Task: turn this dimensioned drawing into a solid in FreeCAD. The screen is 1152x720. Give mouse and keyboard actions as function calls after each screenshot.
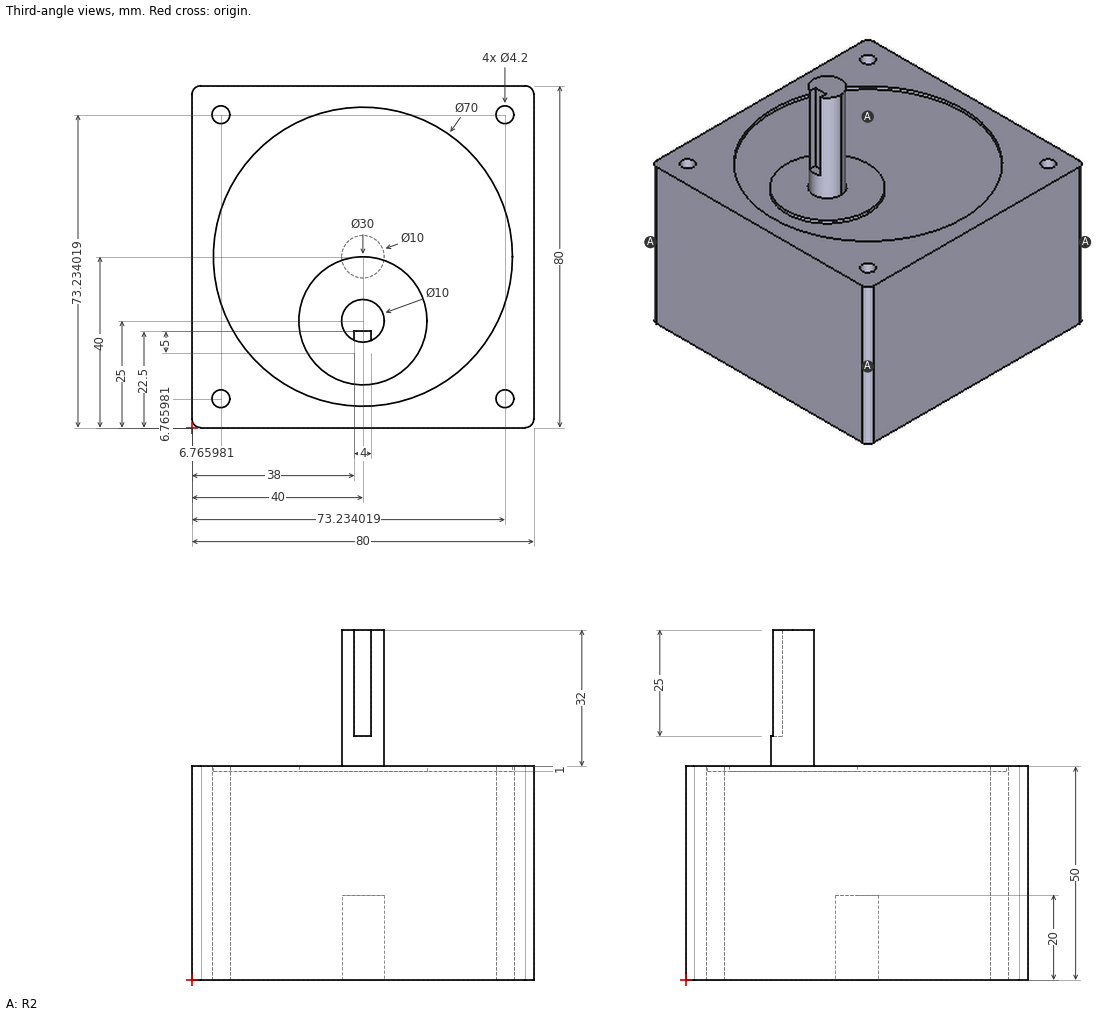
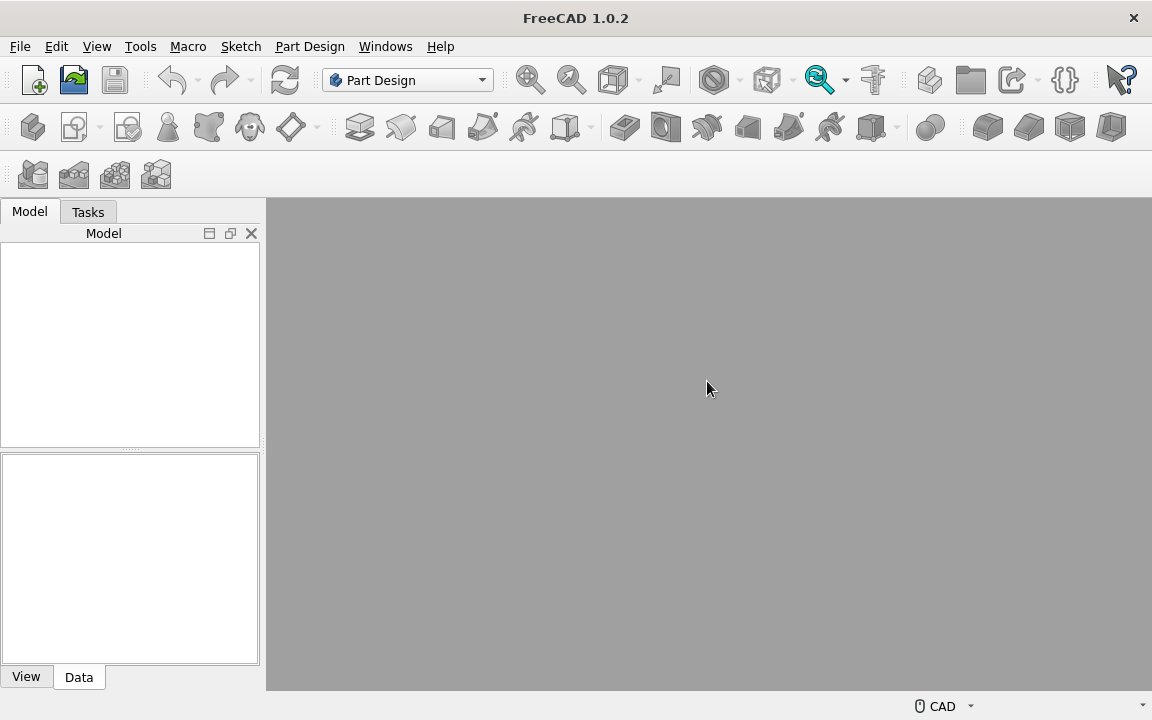
key(ctrl+n)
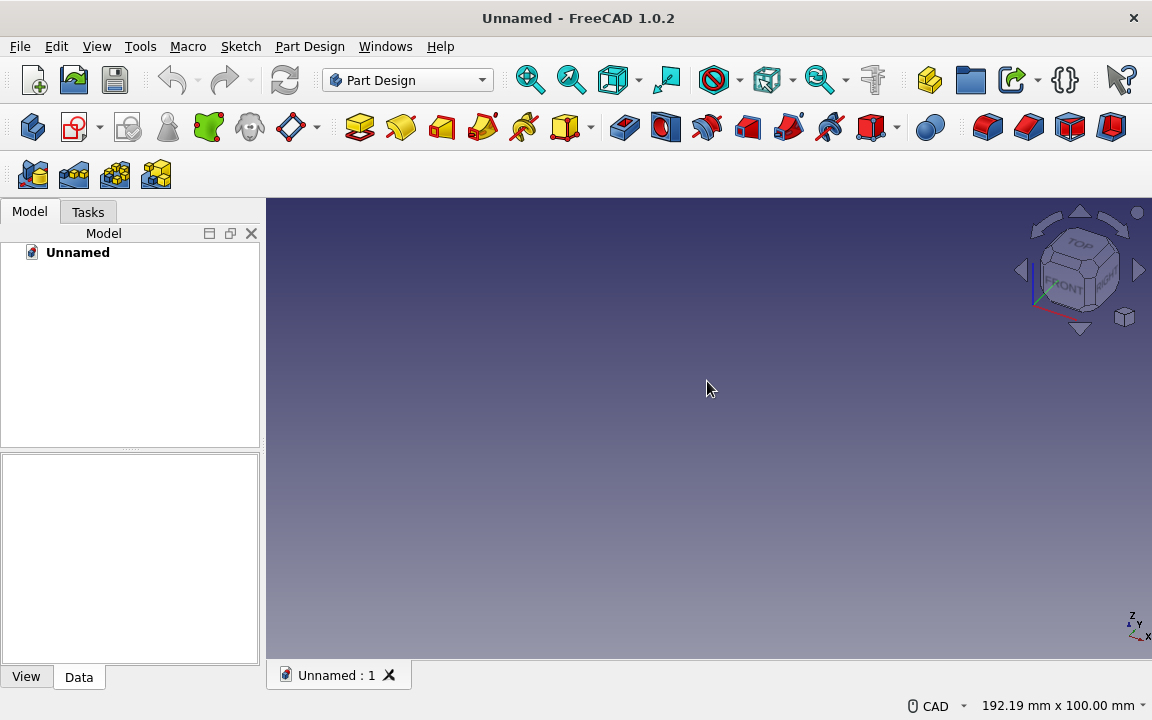
click(74, 128)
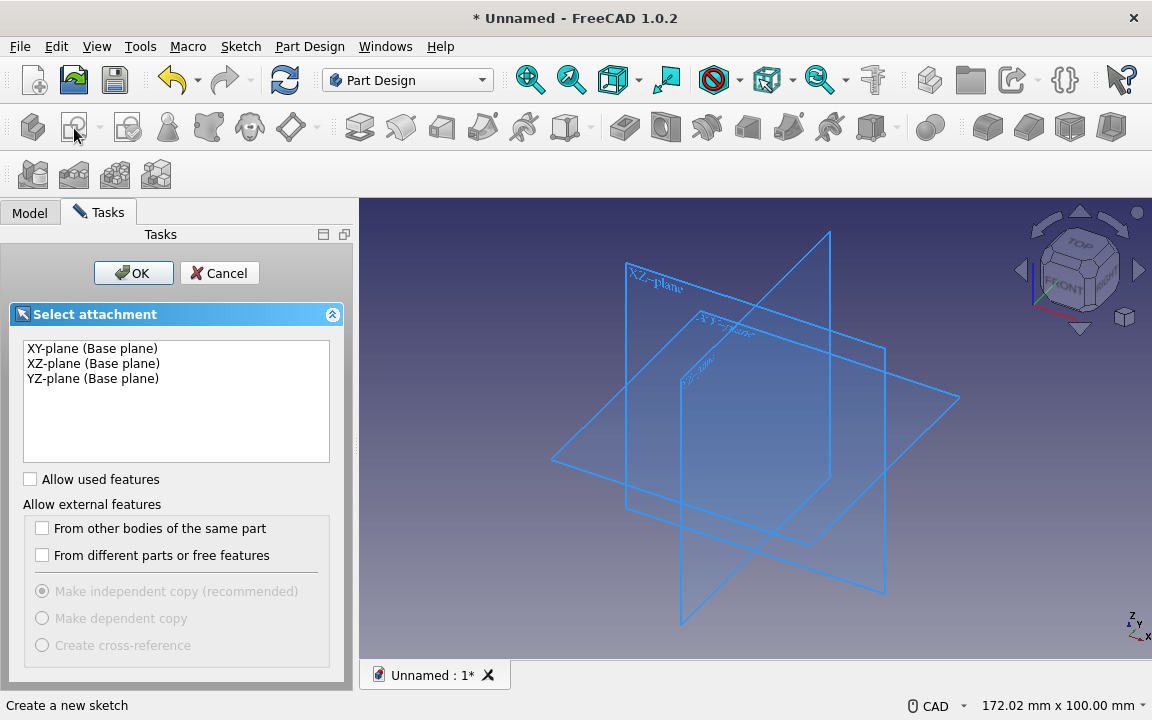
click(84, 348)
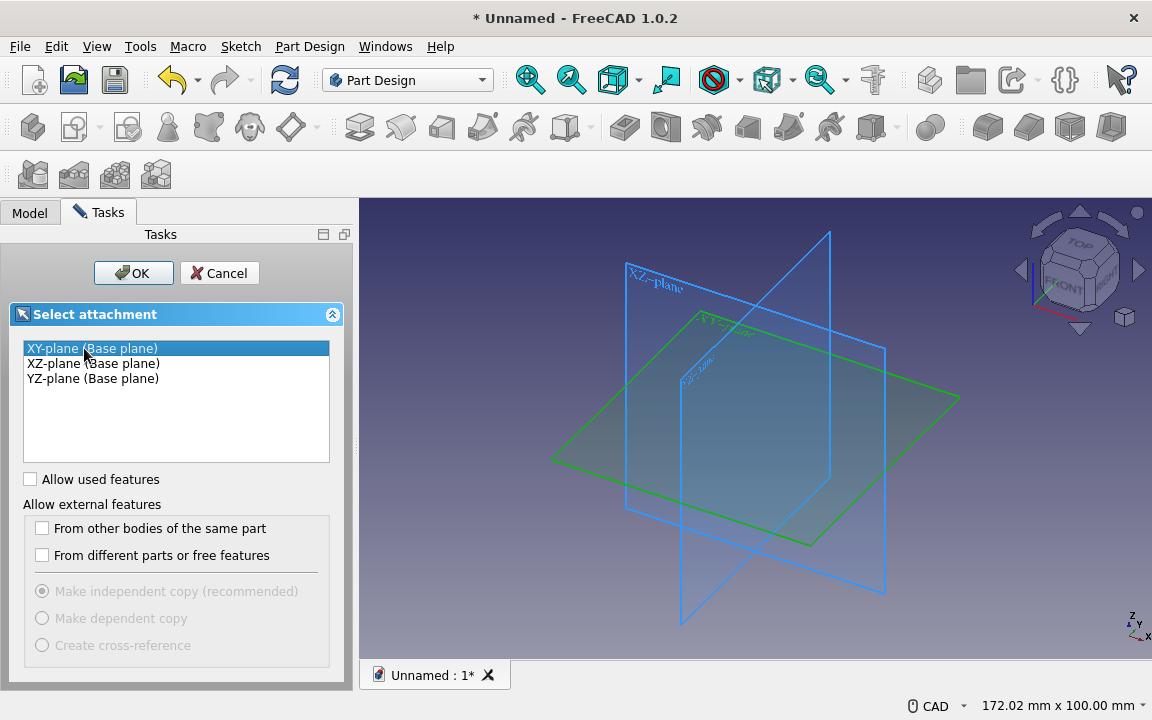
click(134, 273)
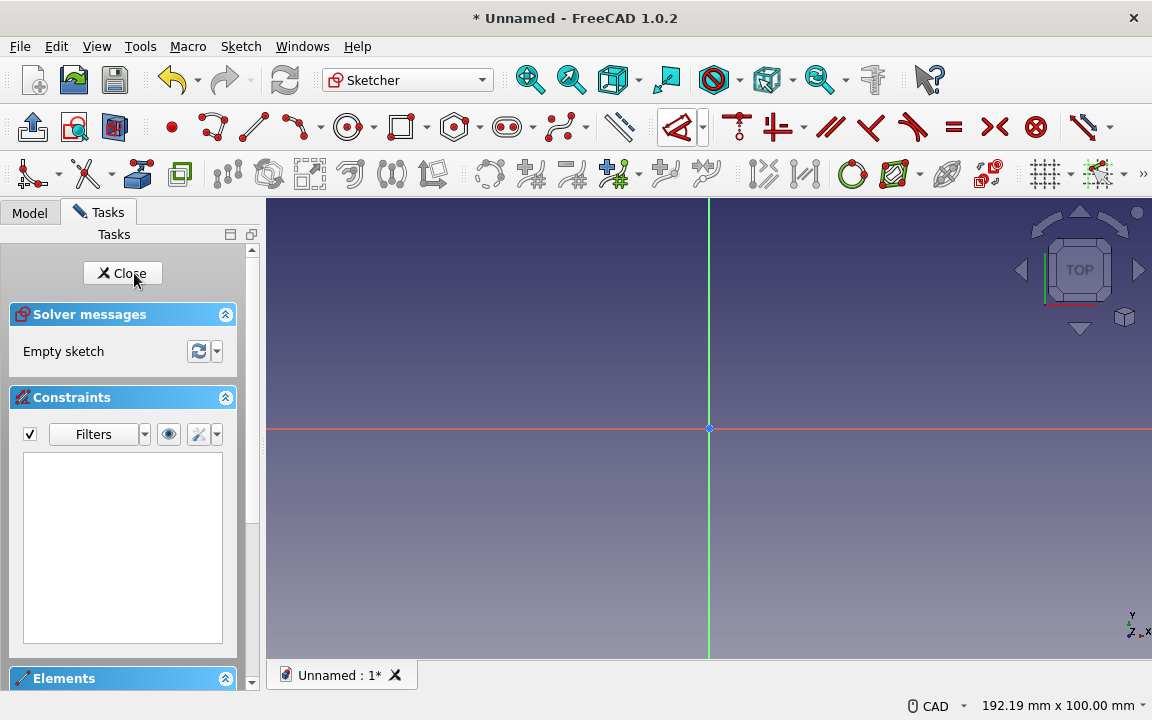
scroll(333, 631, down, 3)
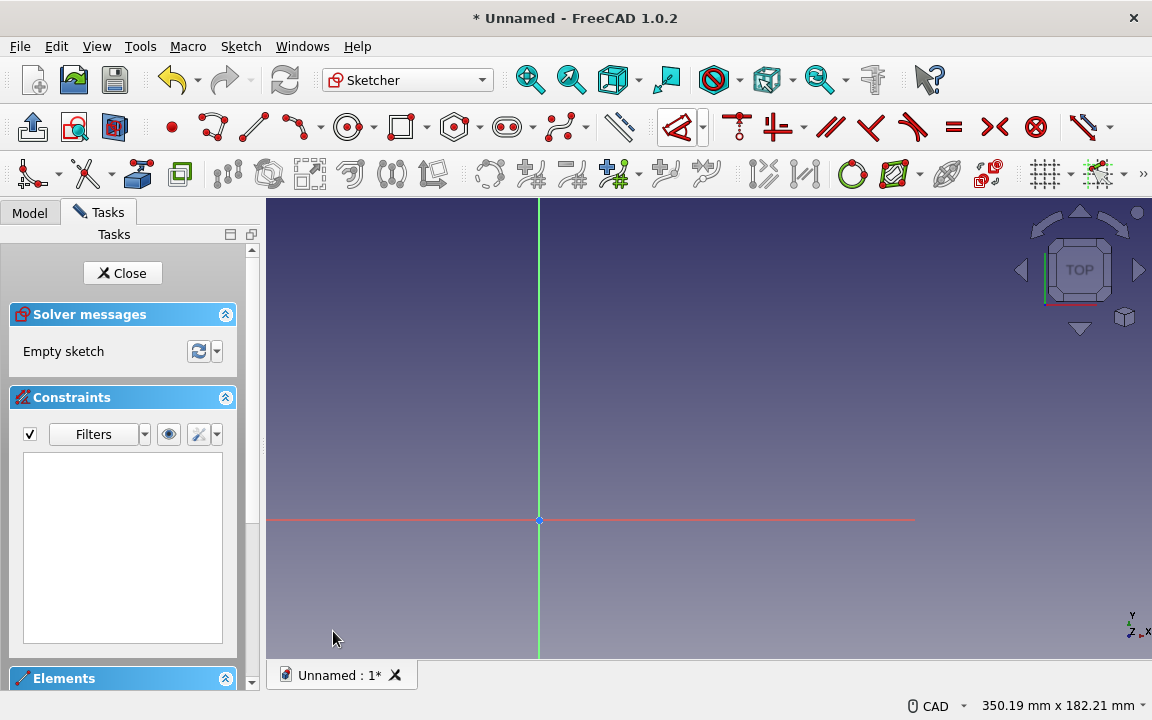
scroll(641, 400, up, 2)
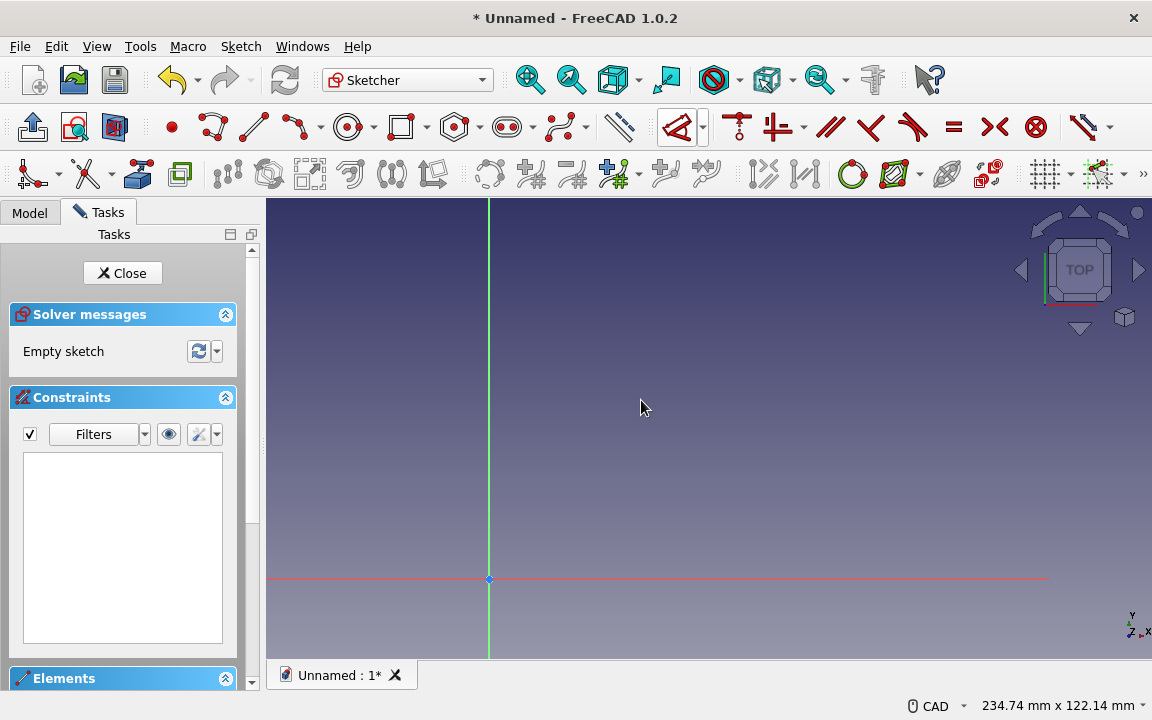
click(400, 128)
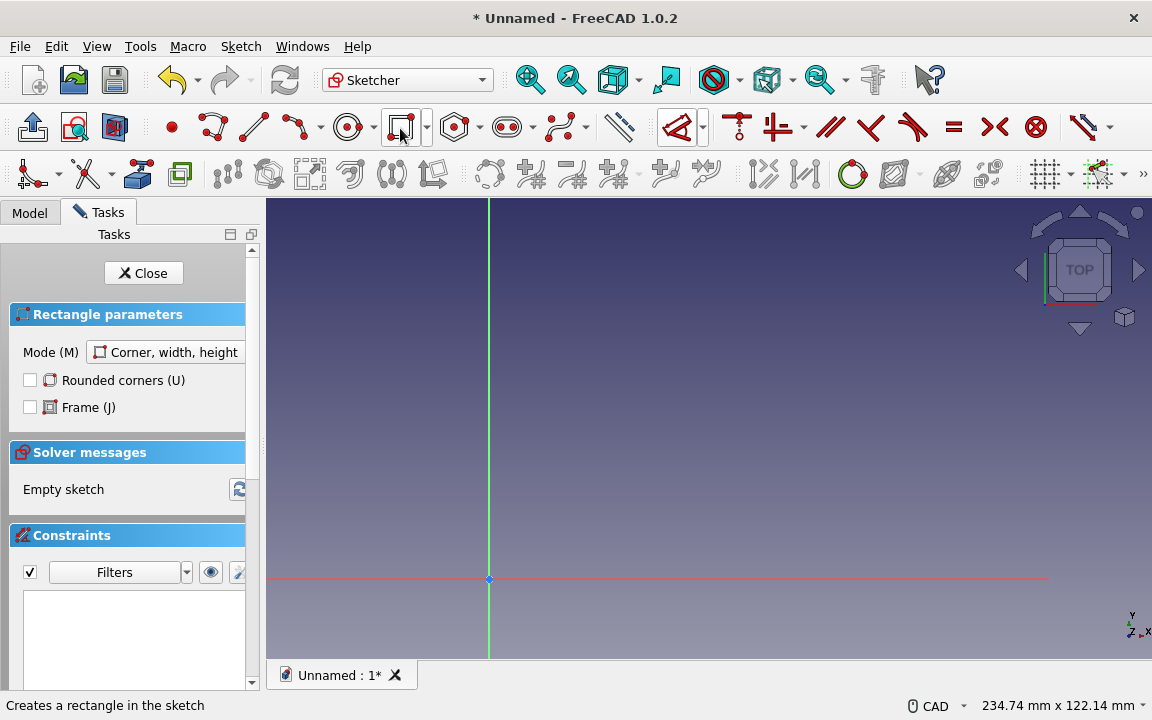
click(489, 579)
click(791, 277)
key(Escape)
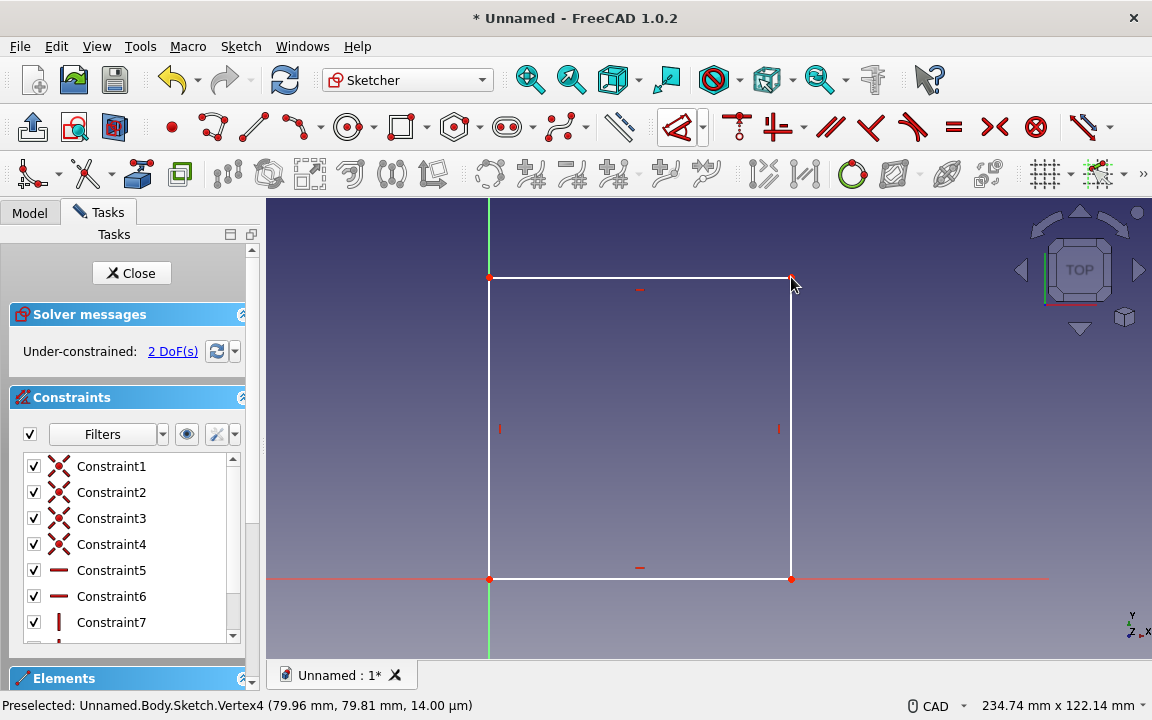
click(580, 579)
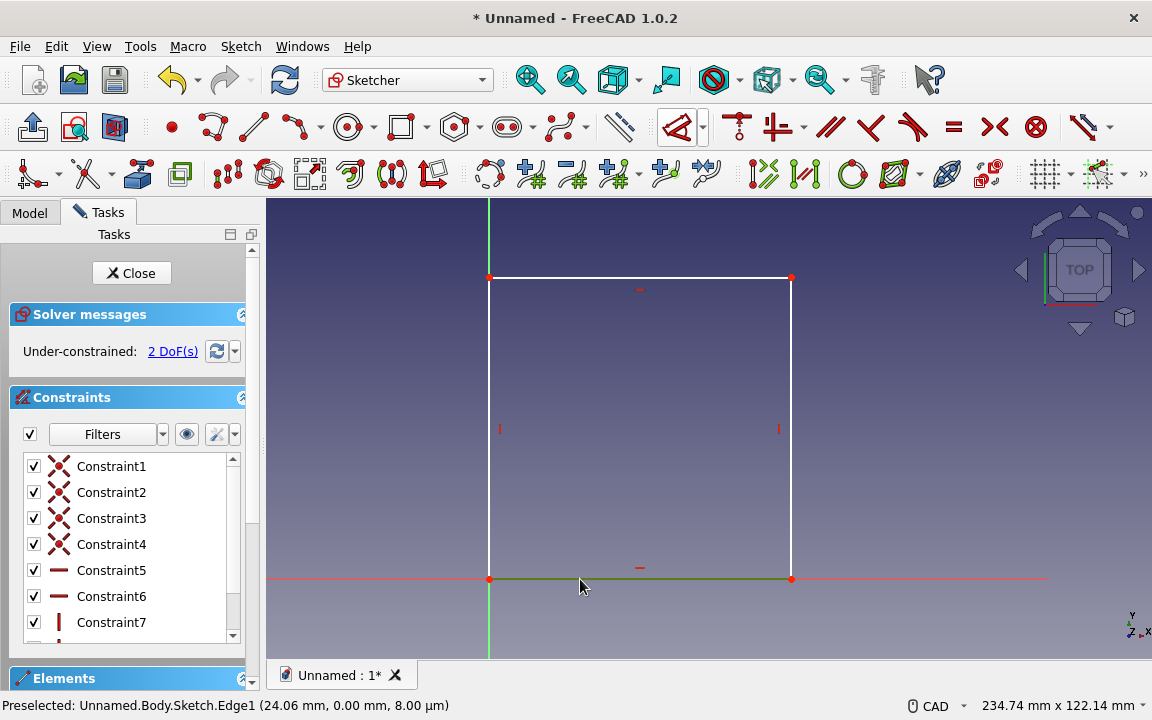
key(l)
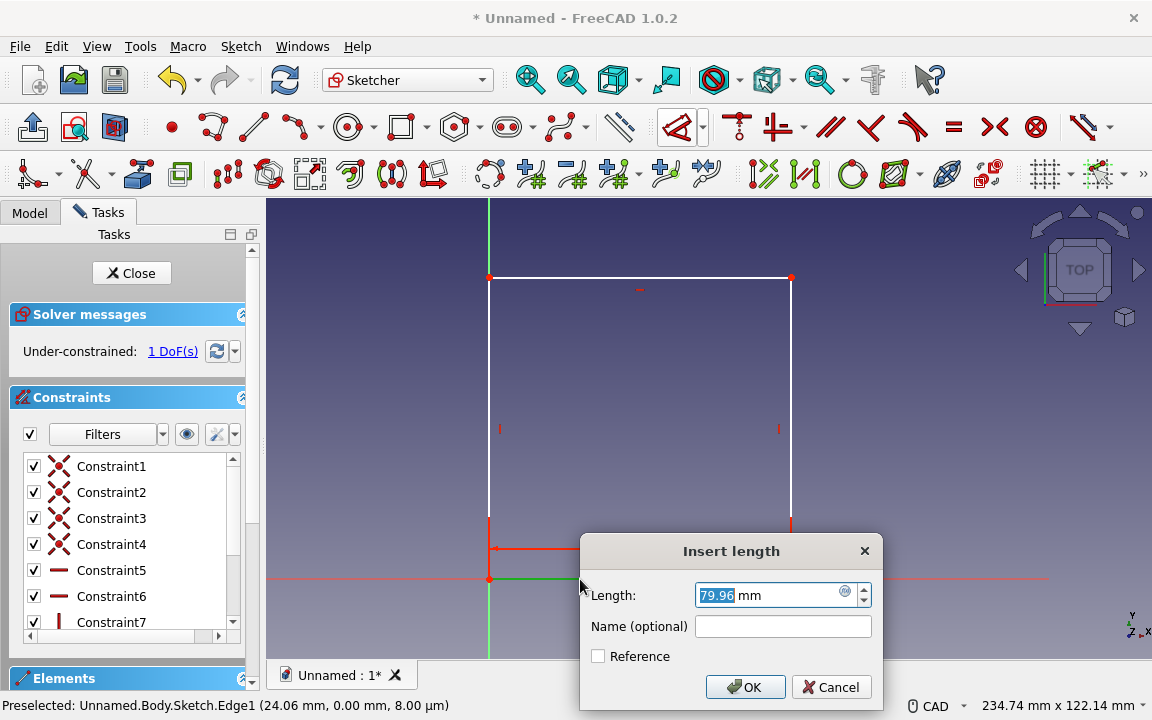
text(80)
key(Return)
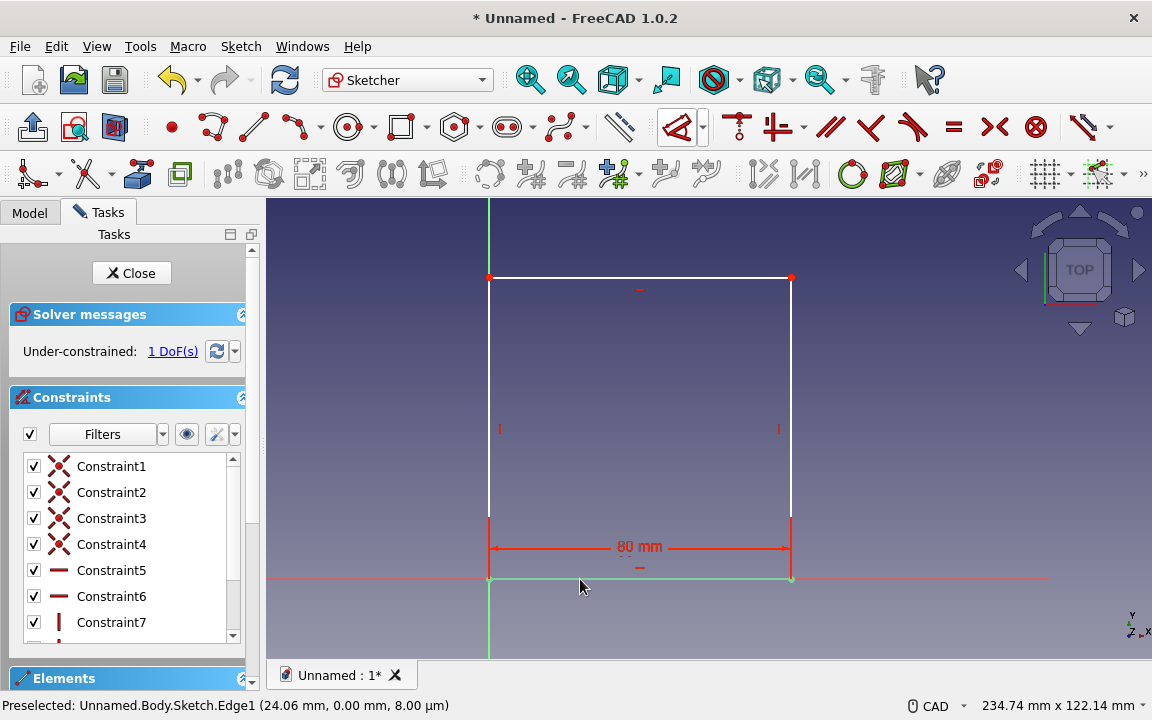
click(791, 489)